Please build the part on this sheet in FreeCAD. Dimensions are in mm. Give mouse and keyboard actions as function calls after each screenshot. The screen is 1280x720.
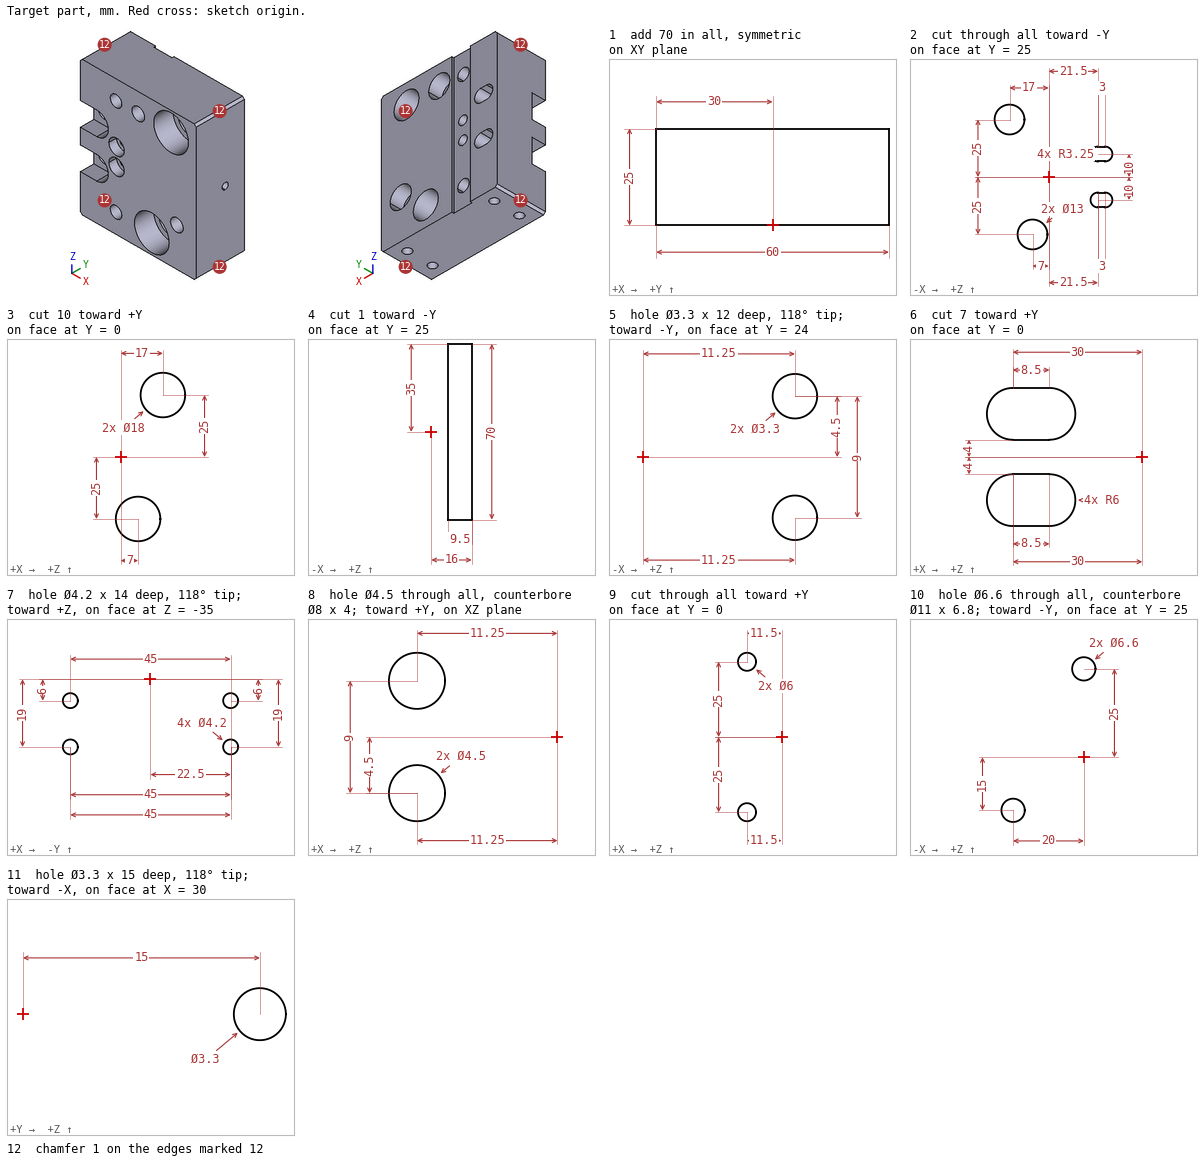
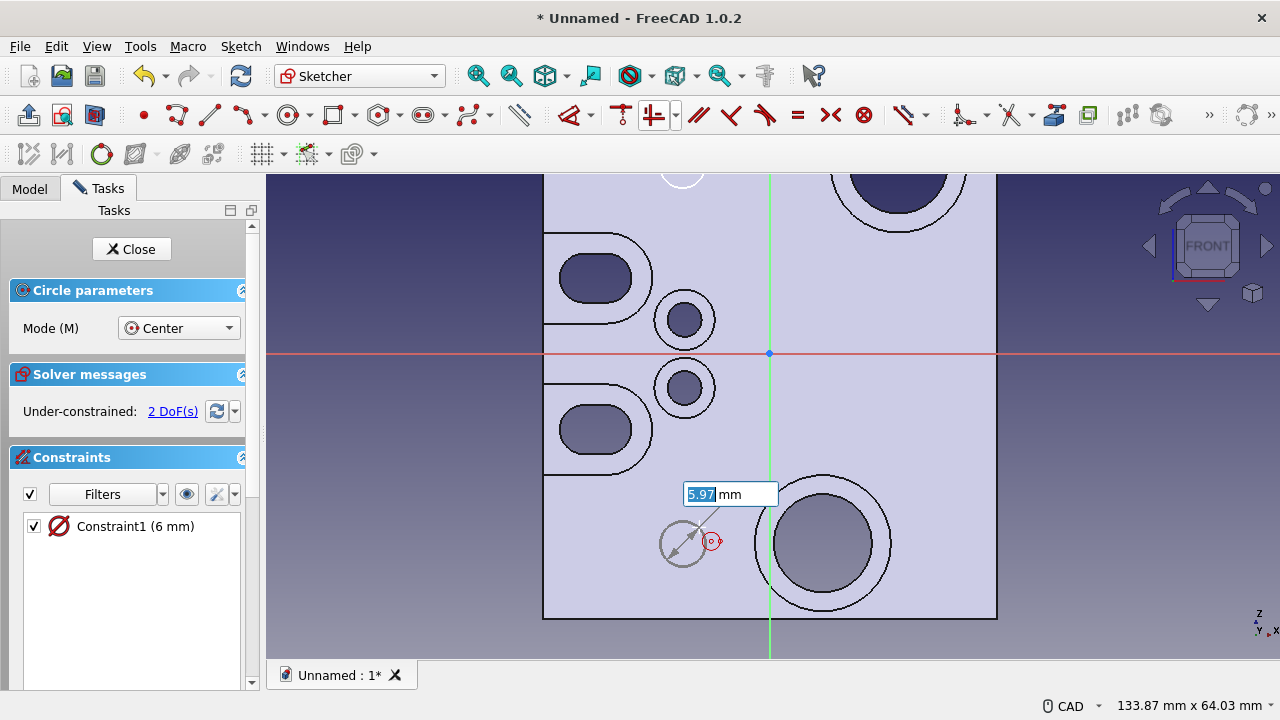
text(6)
key(Return)
key(Escape)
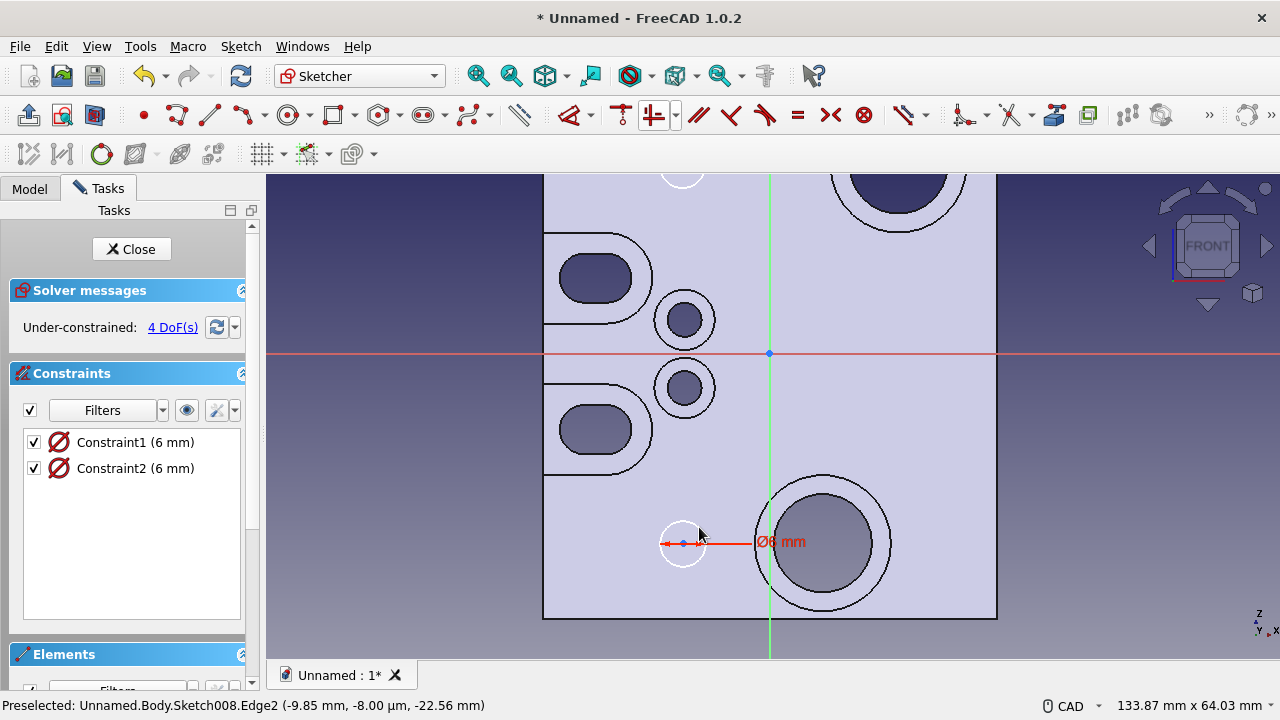
key(d)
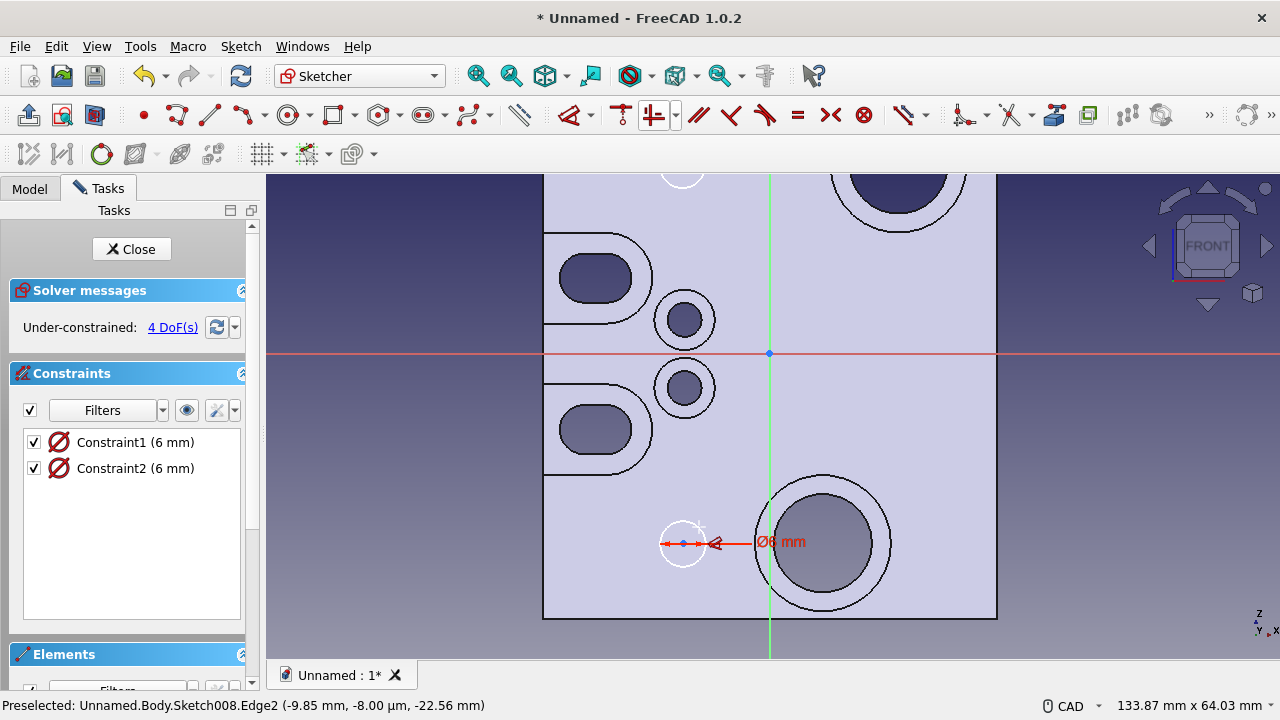
scroll(683, 544, down, 2)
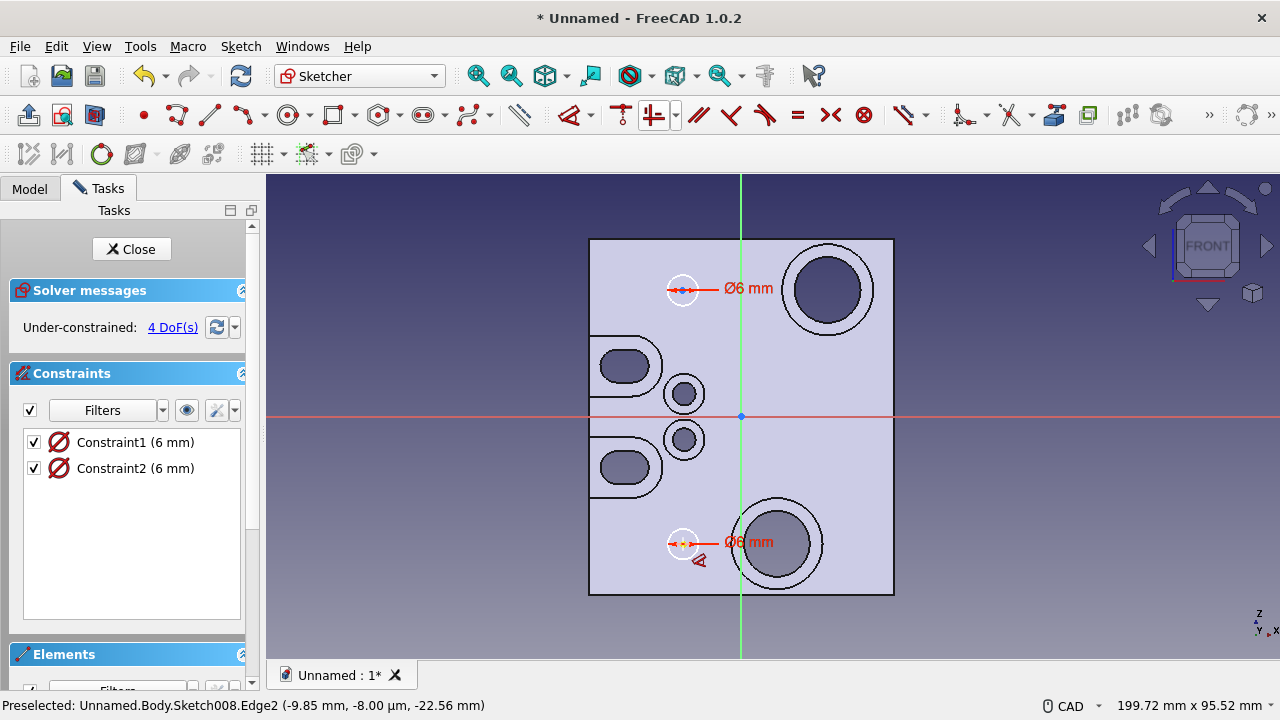
click(683, 290)
click(775, 354)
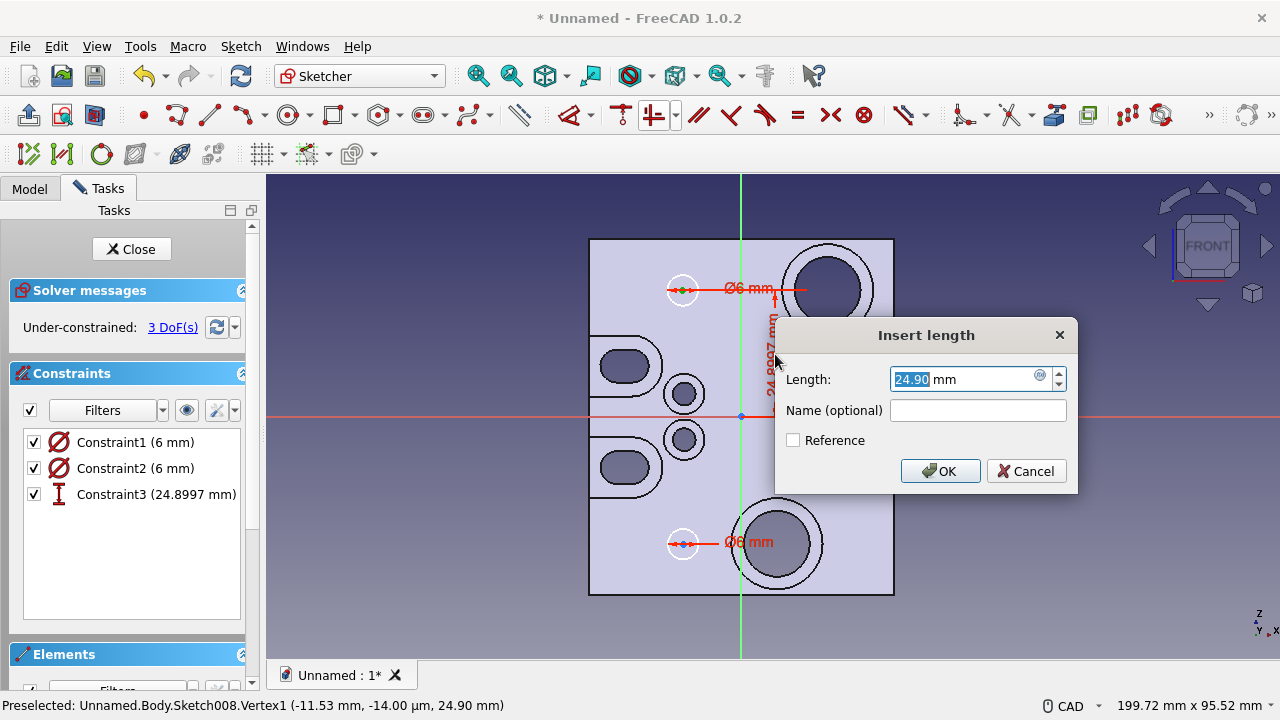
text(25)
key(Return)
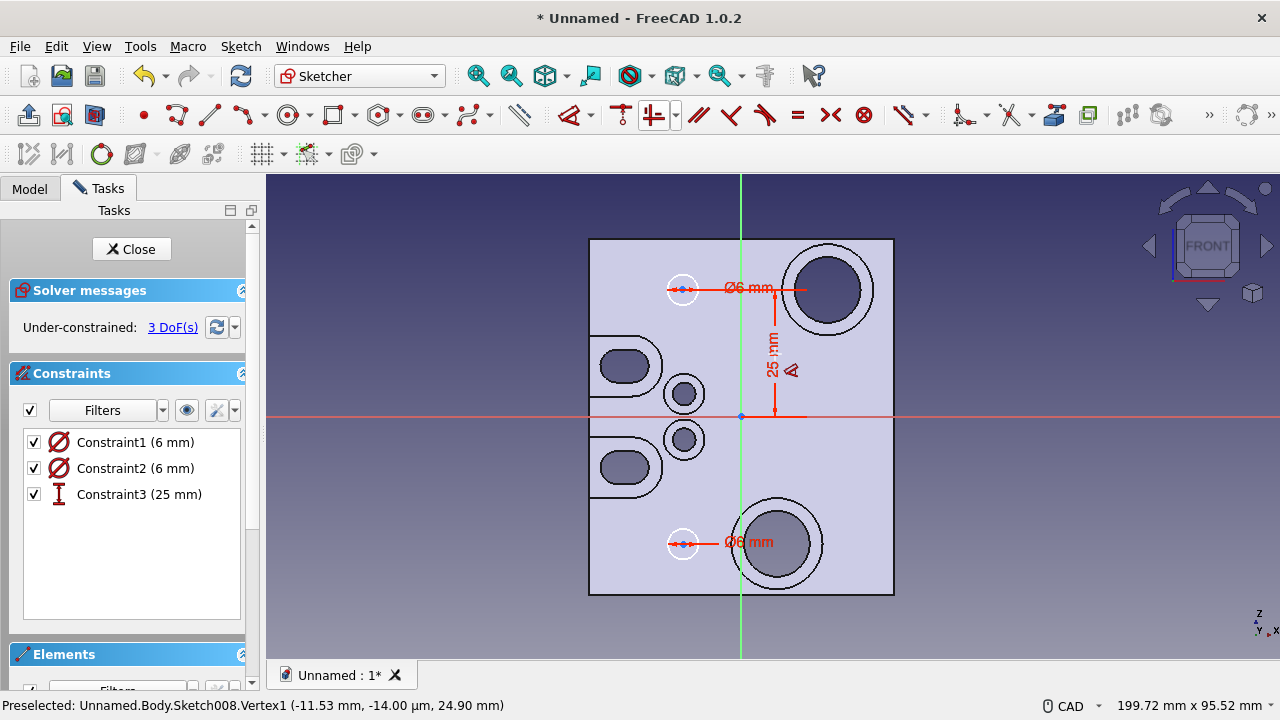
click(683, 544)
click(775, 481)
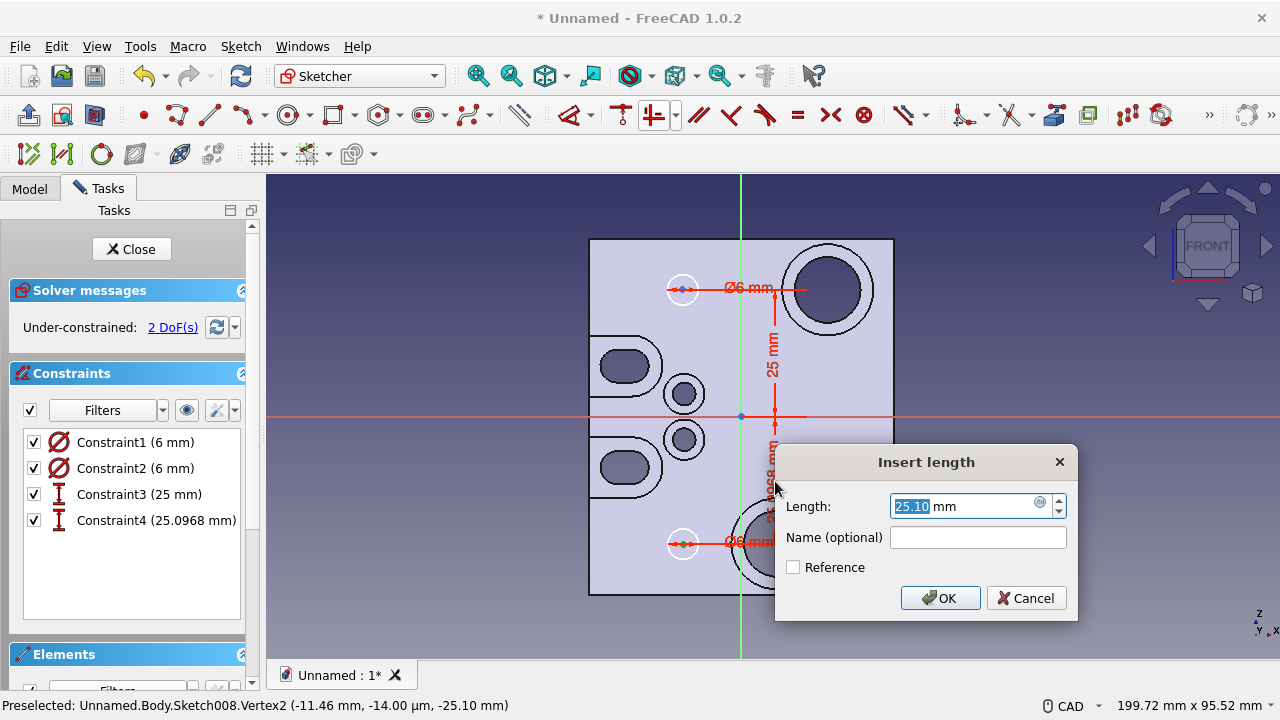
text(25)
key(Return)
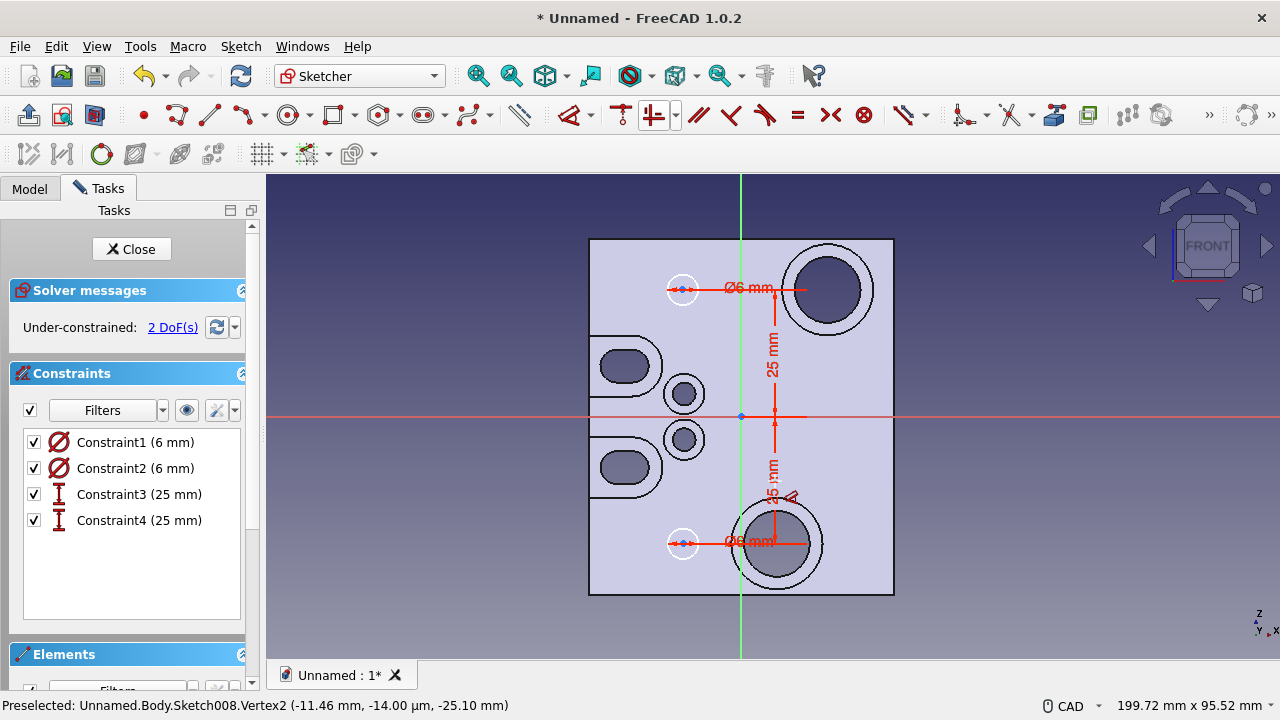
click(683, 290)
click(712, 256)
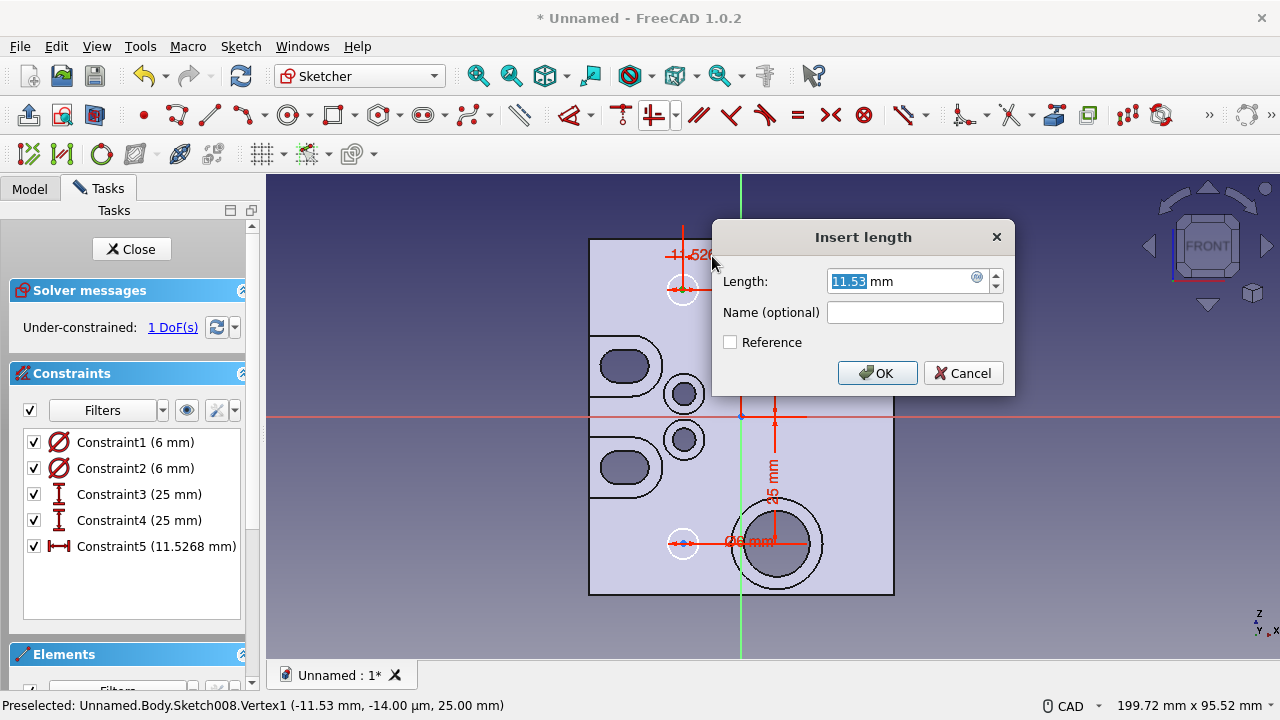
text(11.5)
key(Return)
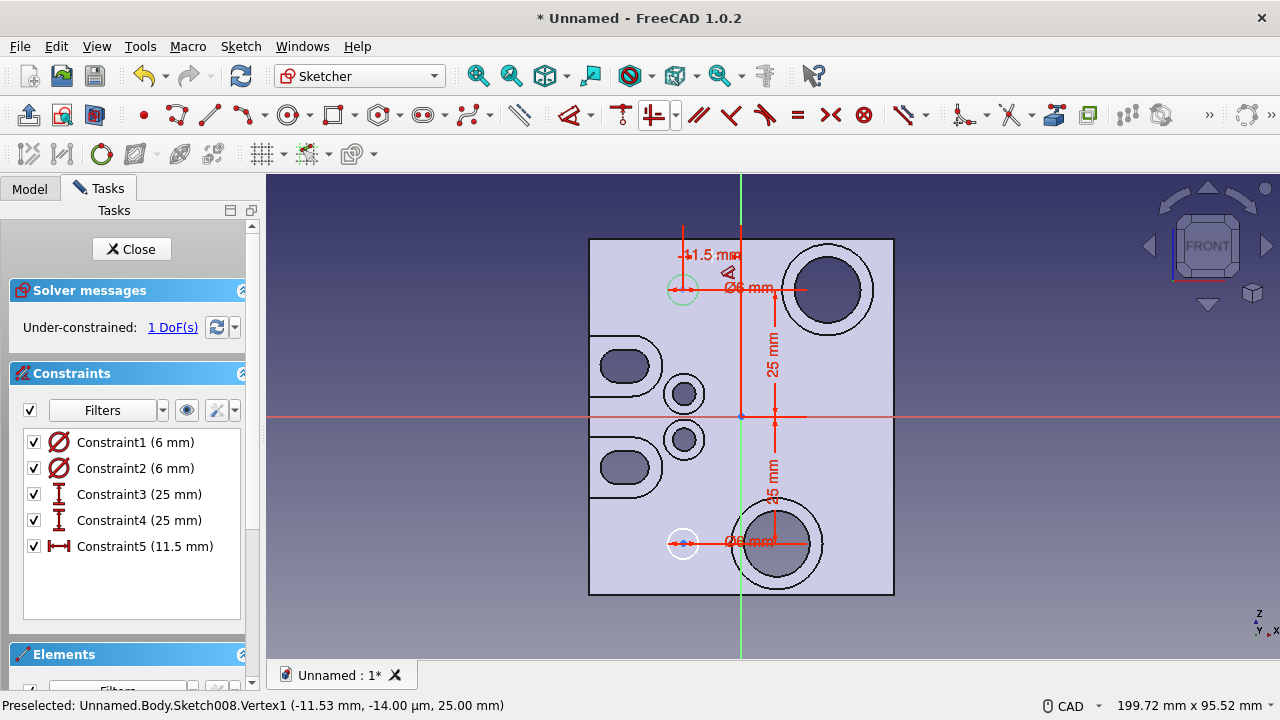
click(683, 544)
click(712, 578)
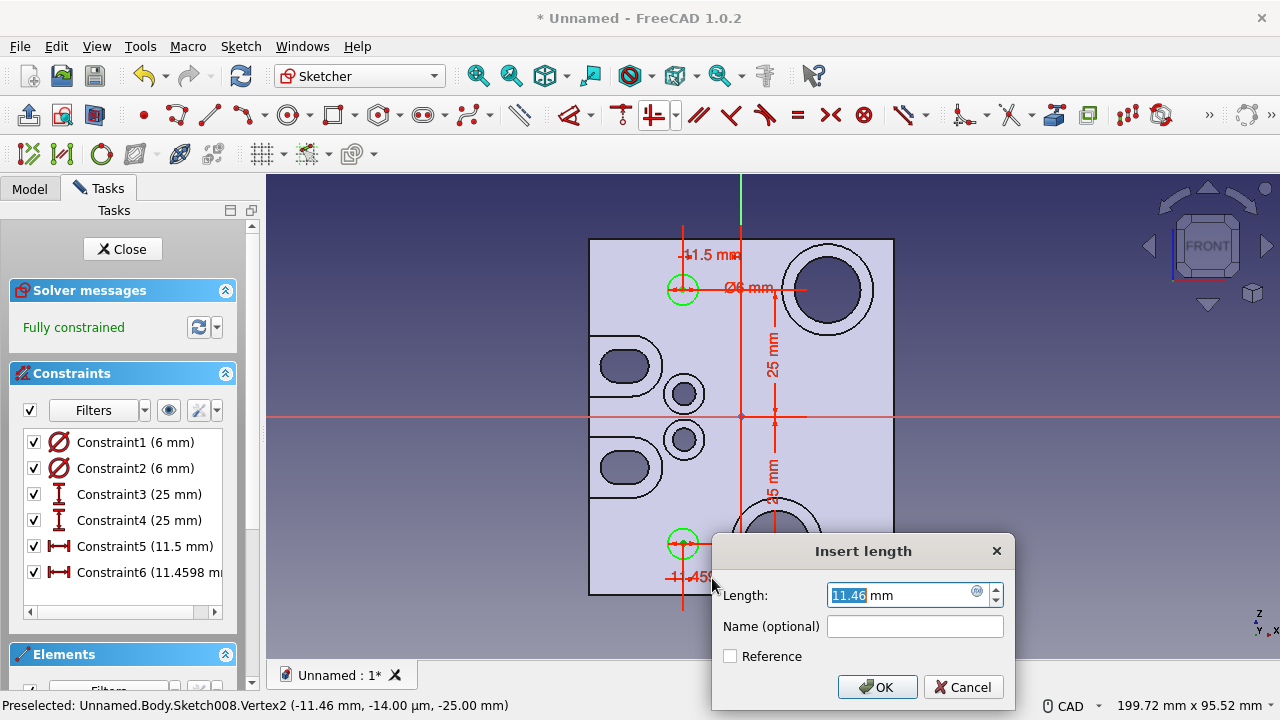
text(11.5)
key(Return)
key(Escape)